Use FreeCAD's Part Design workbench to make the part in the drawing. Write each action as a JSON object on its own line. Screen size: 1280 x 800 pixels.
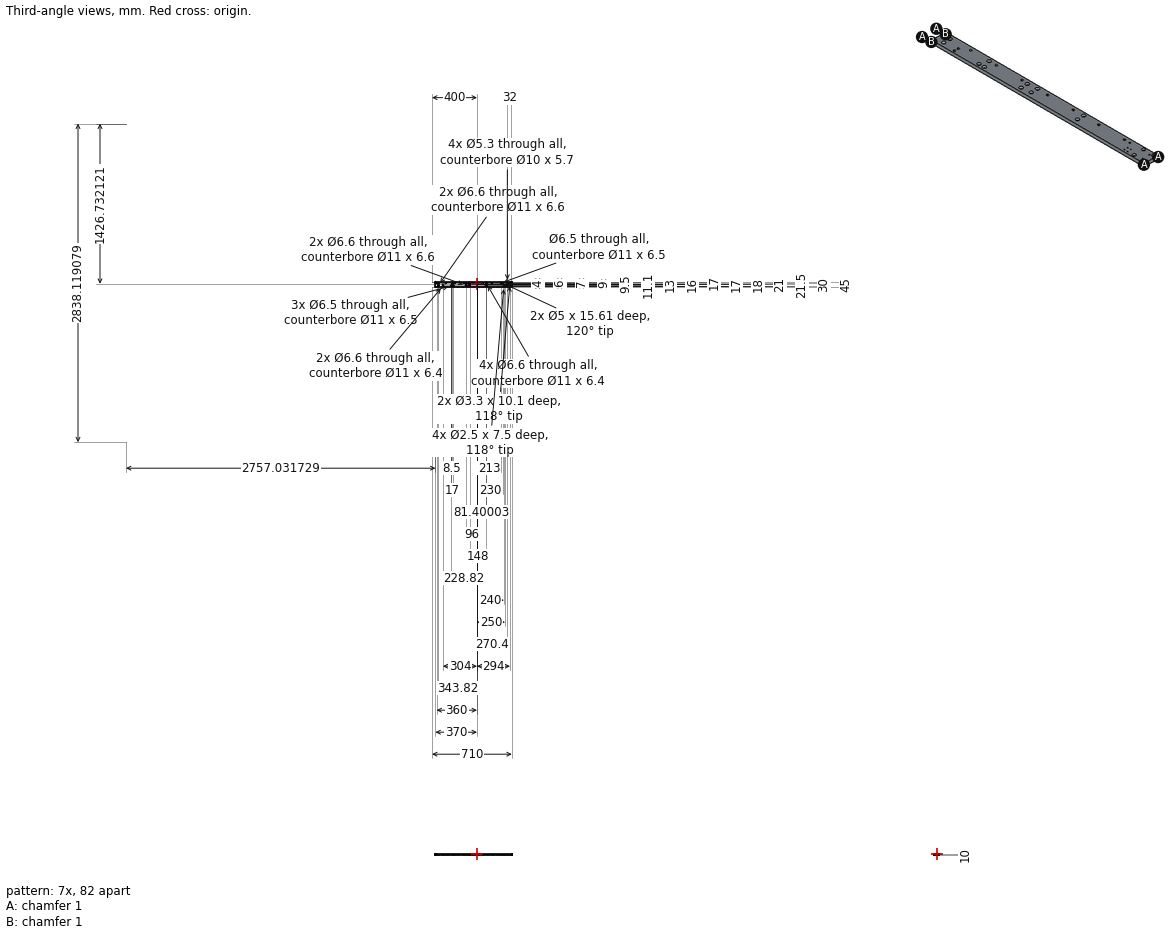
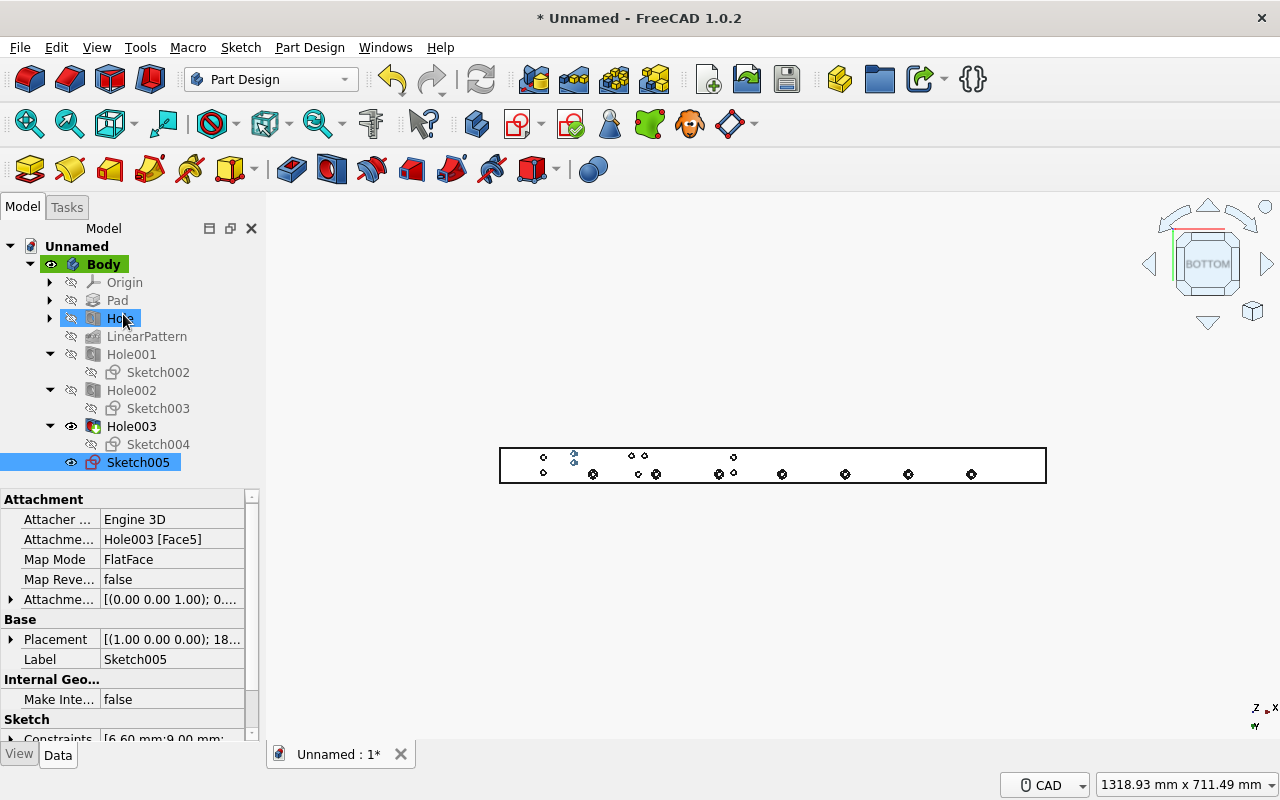
{"action": "left_click", "coordinate": [332, 170]}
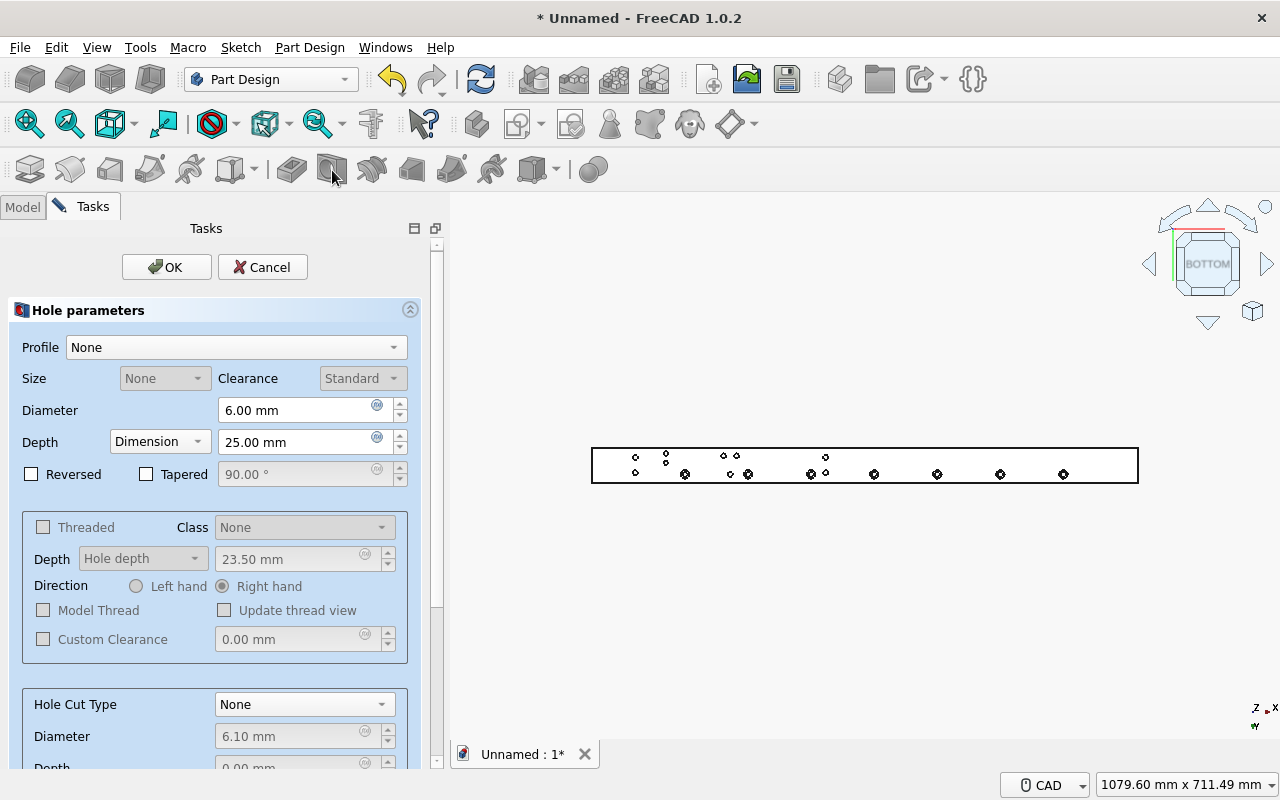
{"action": "triple_click", "coordinate": [305, 410]}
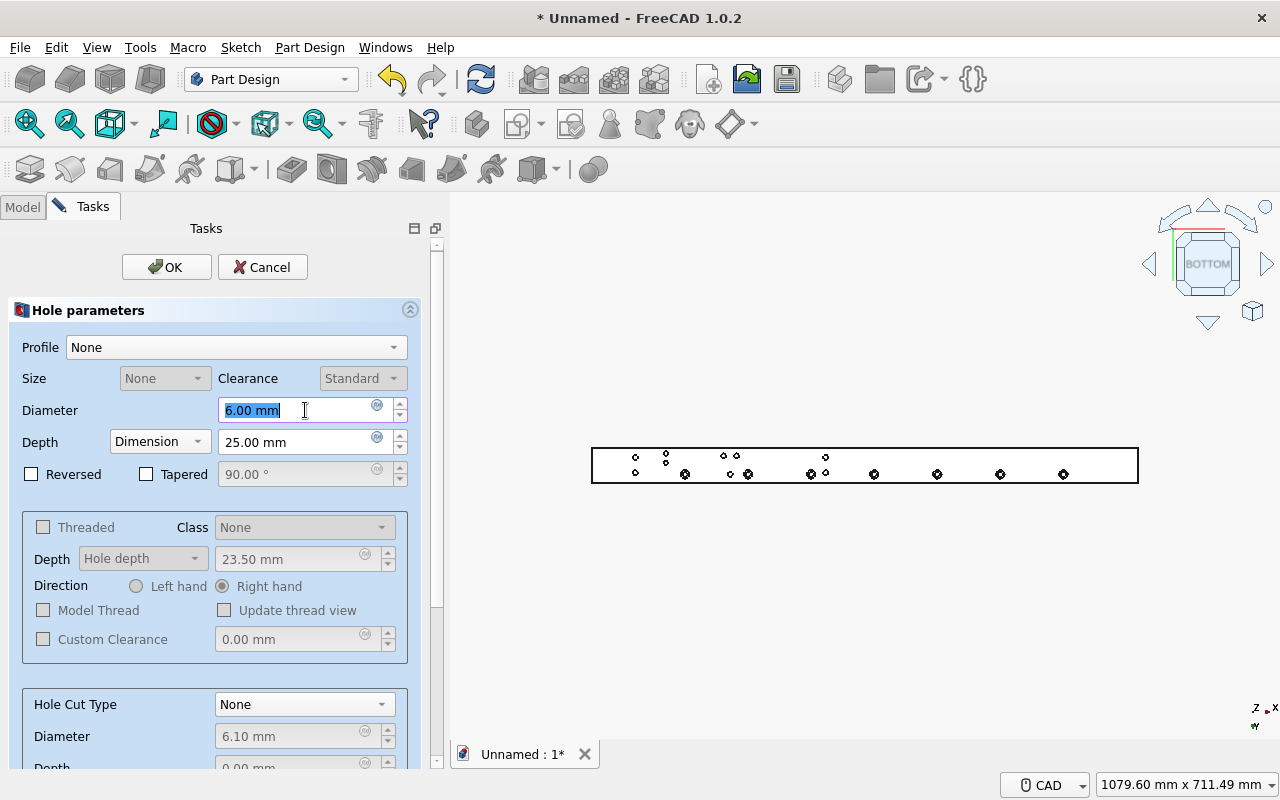
{"action": "type", "text": "6.6"}
{"action": "key", "text": "Tab"}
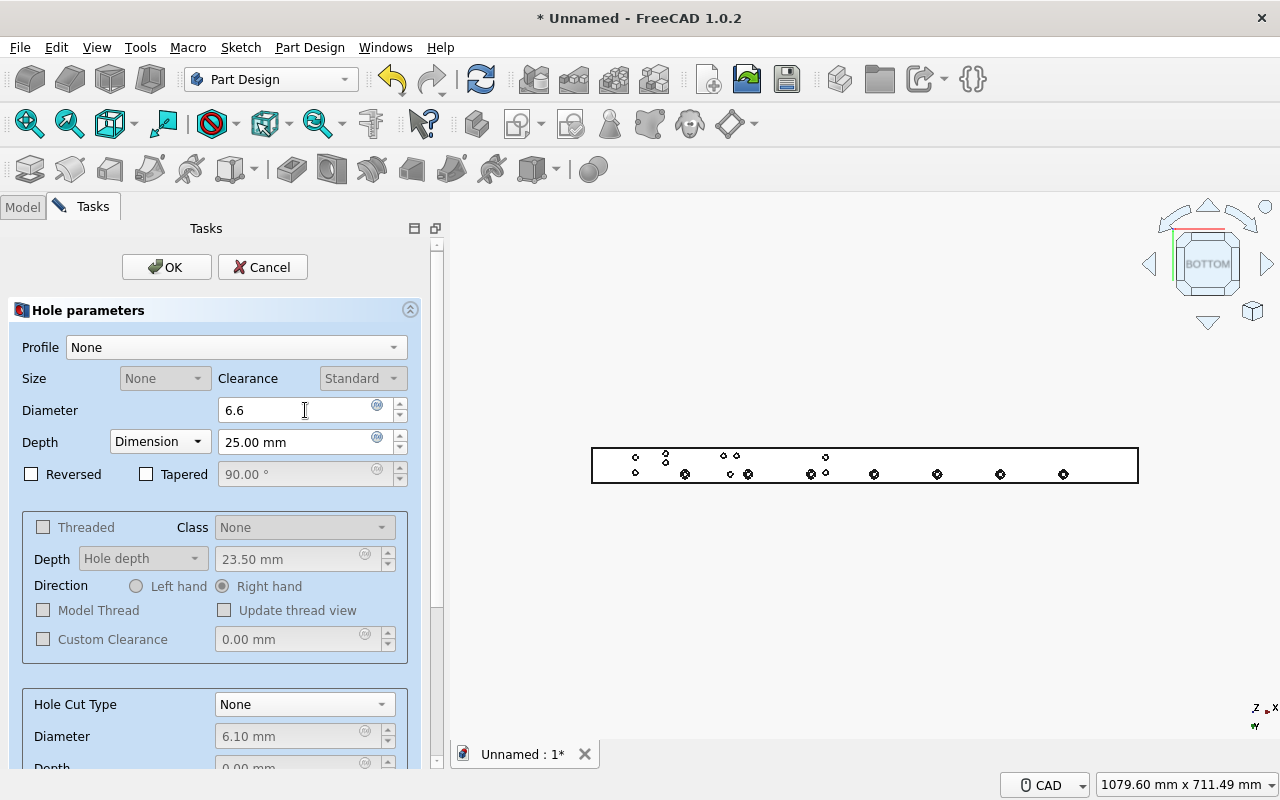
{"action": "left_click", "coordinate": [161, 442]}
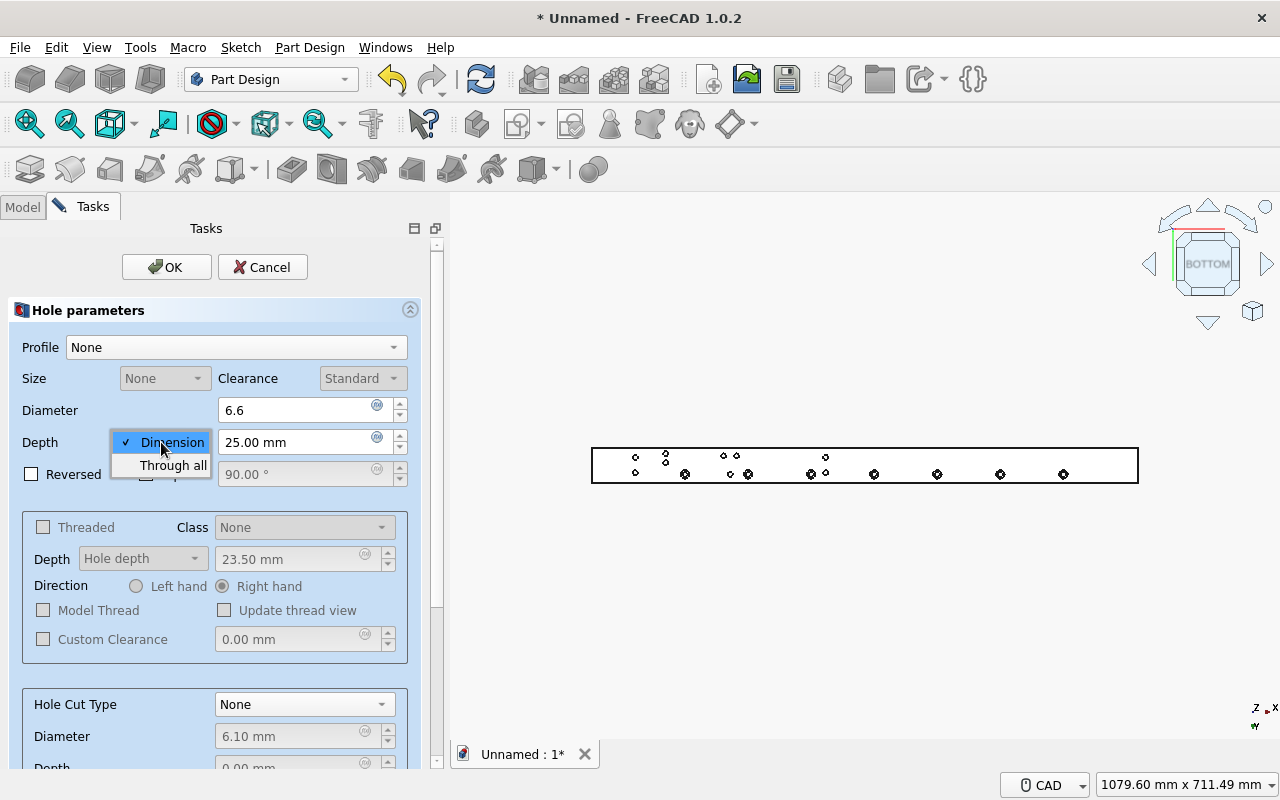
{"action": "left_click", "coordinate": [160, 466]}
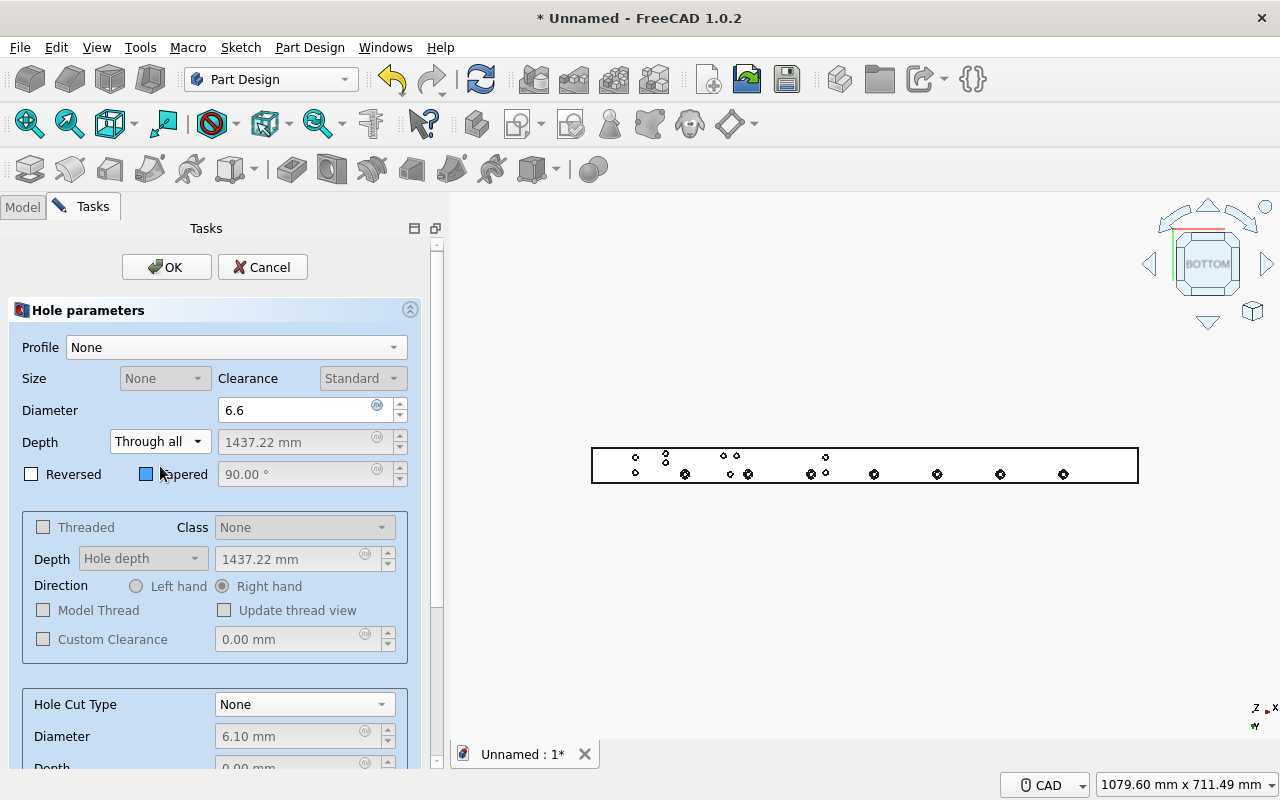
{"action": "left_click", "coordinate": [306, 704]}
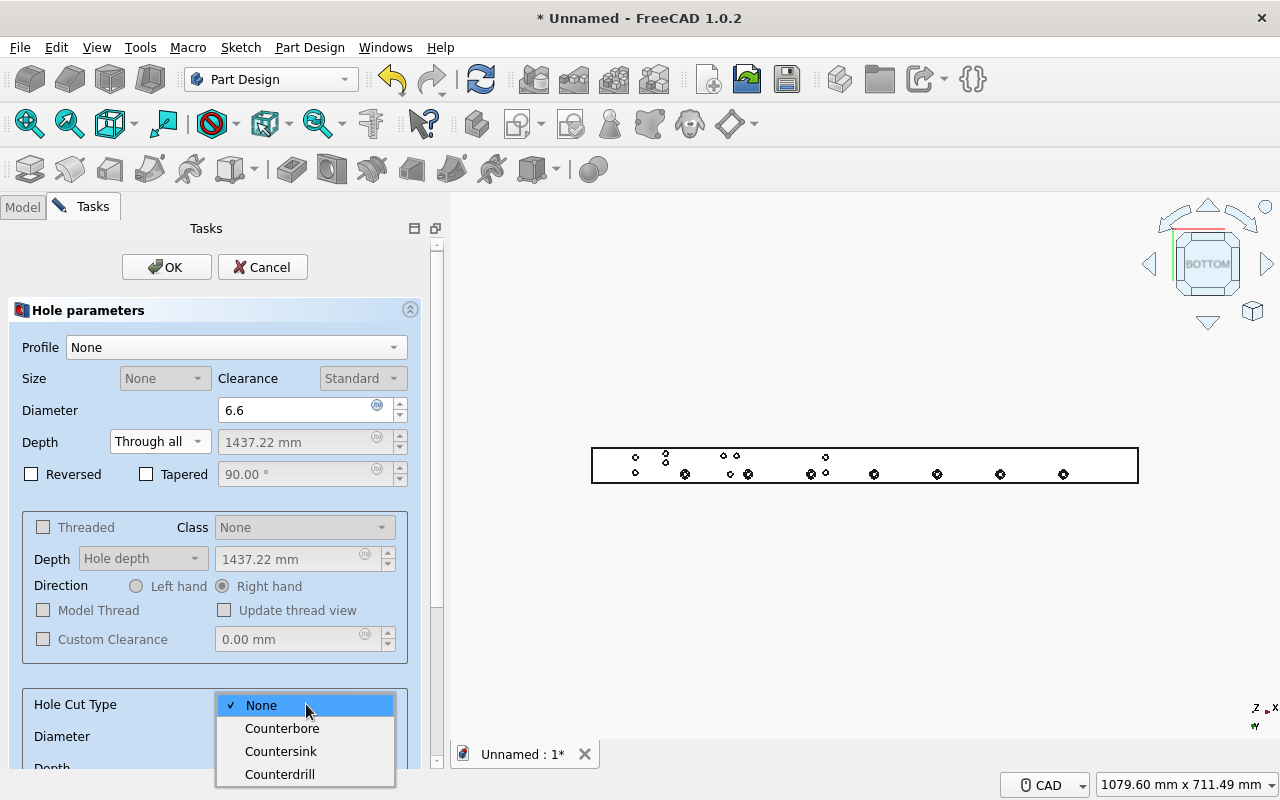
{"action": "left_click", "coordinate": [304, 728]}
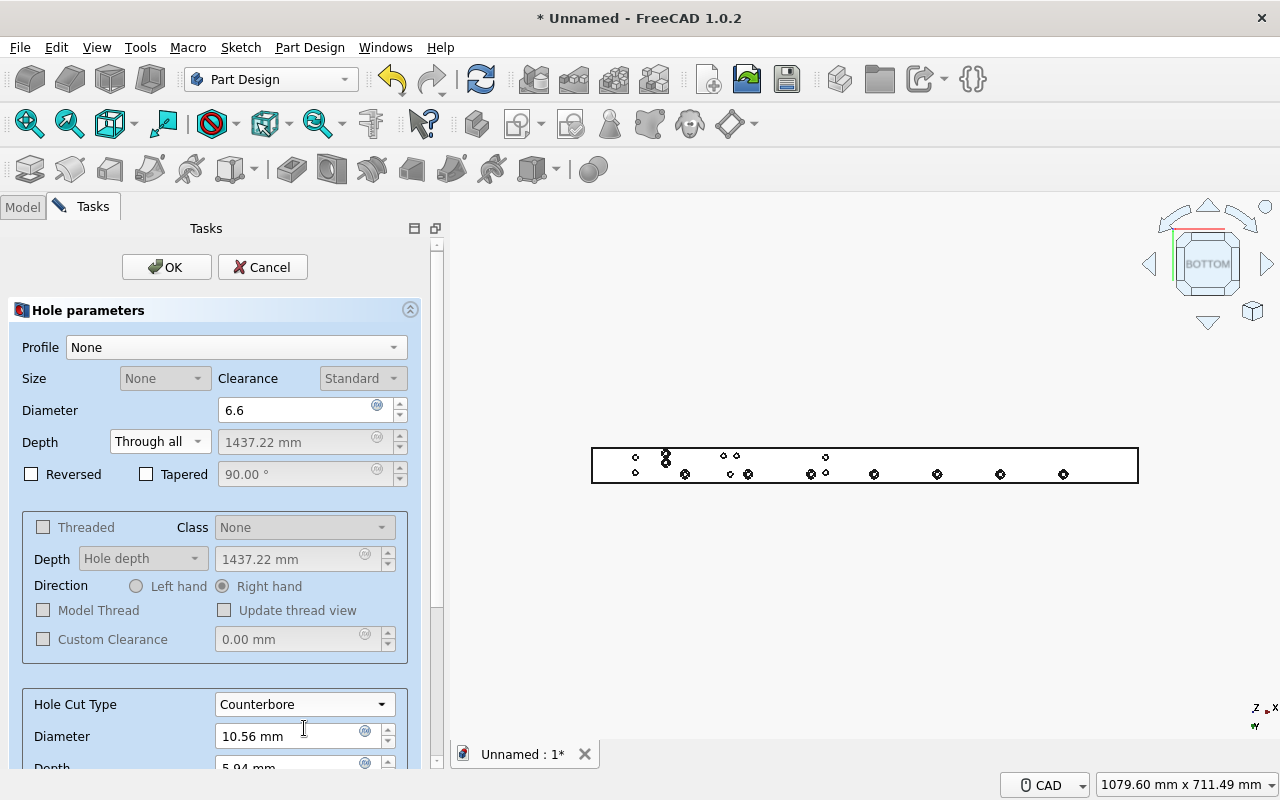
{"action": "triple_click", "coordinate": [298, 736]}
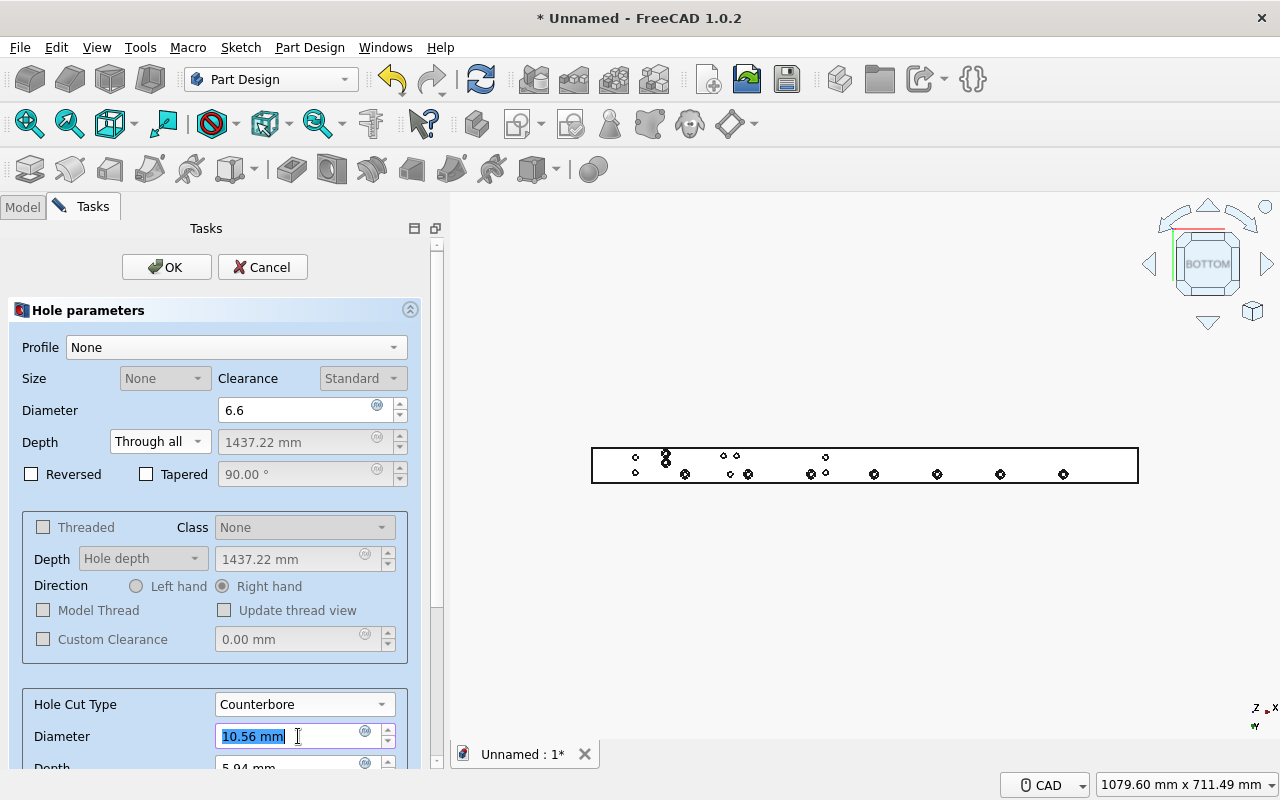
{"action": "type", "text": "11"}
{"action": "key", "text": "Tab"}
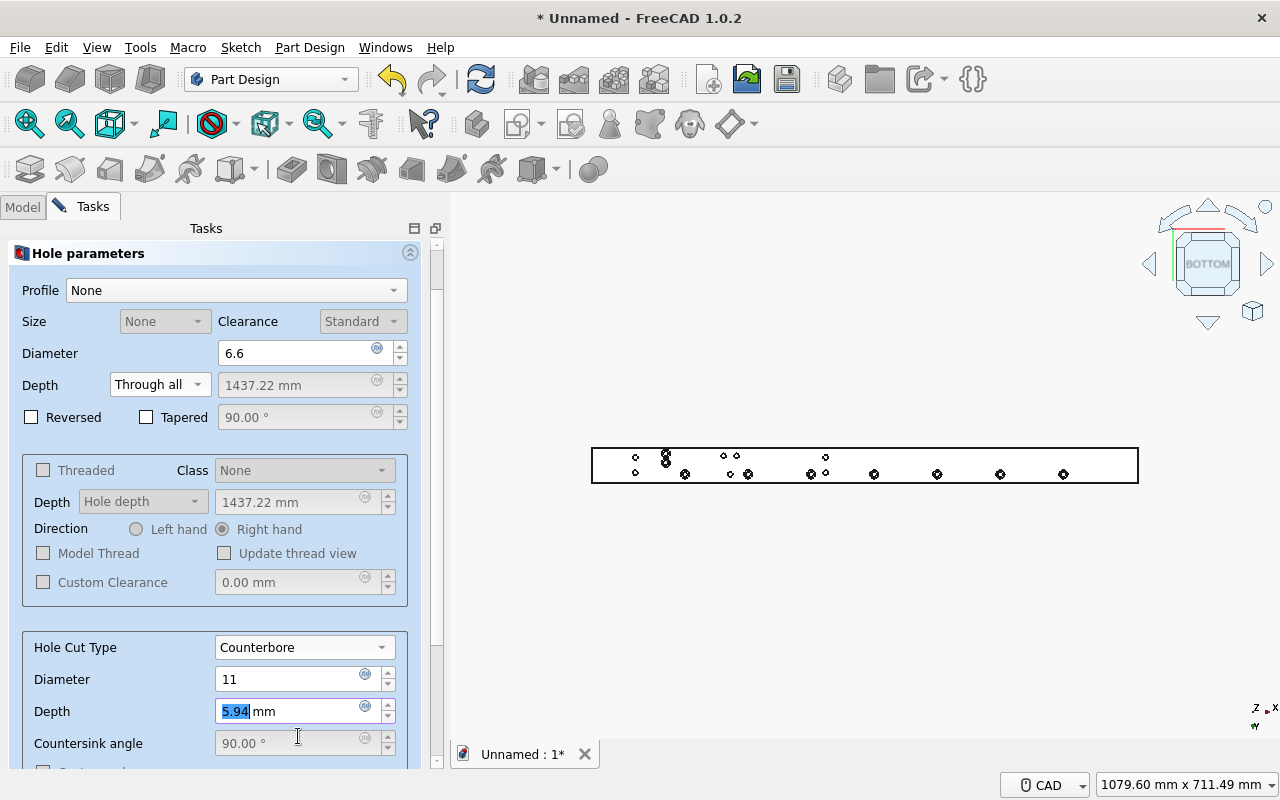
{"action": "type", "text": "6.4"}
{"action": "key", "text": "Tab"}